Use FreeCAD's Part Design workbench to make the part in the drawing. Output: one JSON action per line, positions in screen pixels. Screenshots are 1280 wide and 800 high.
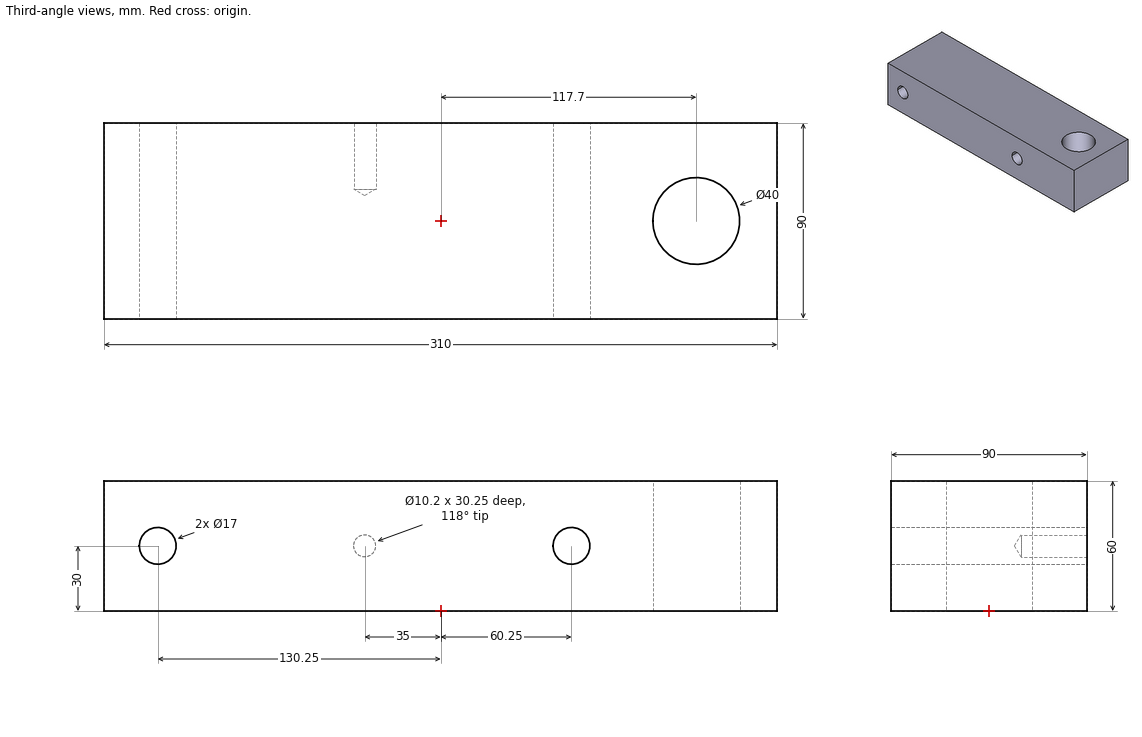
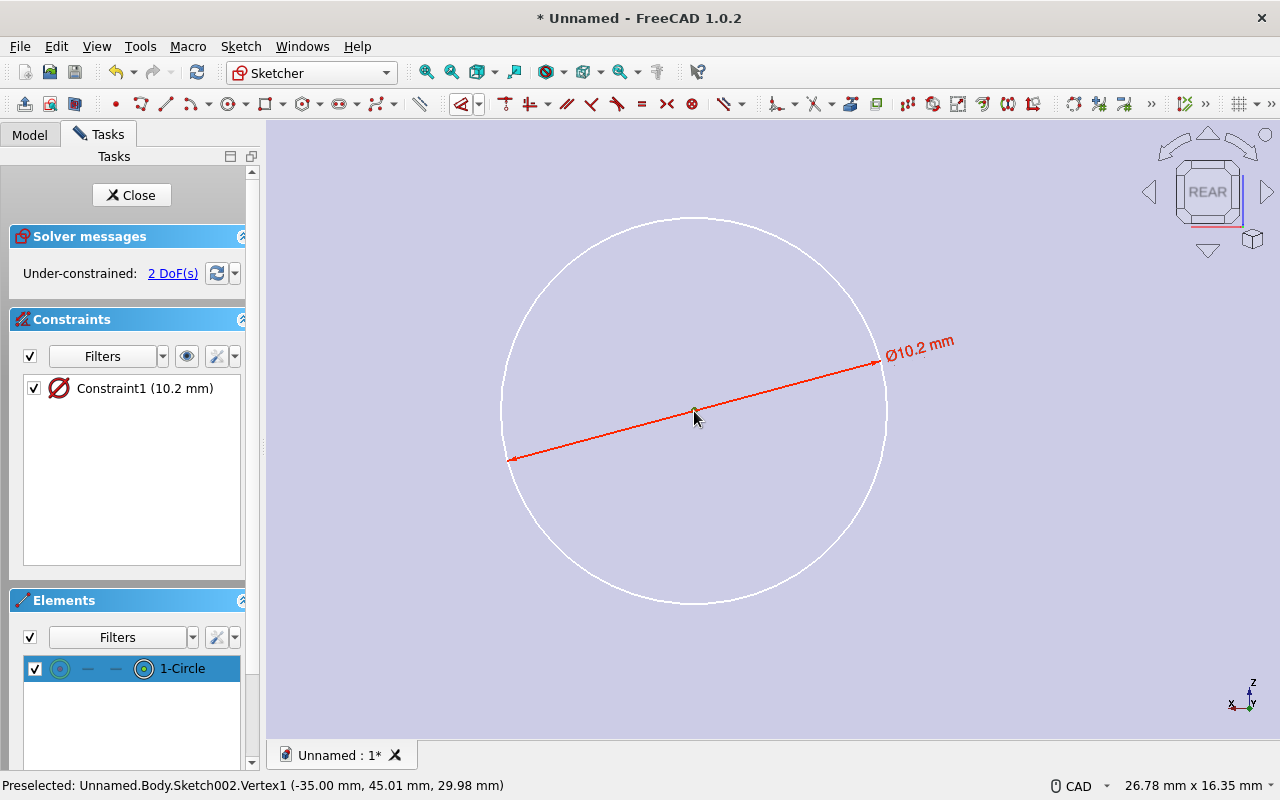
{"action": "key", "text": "l"}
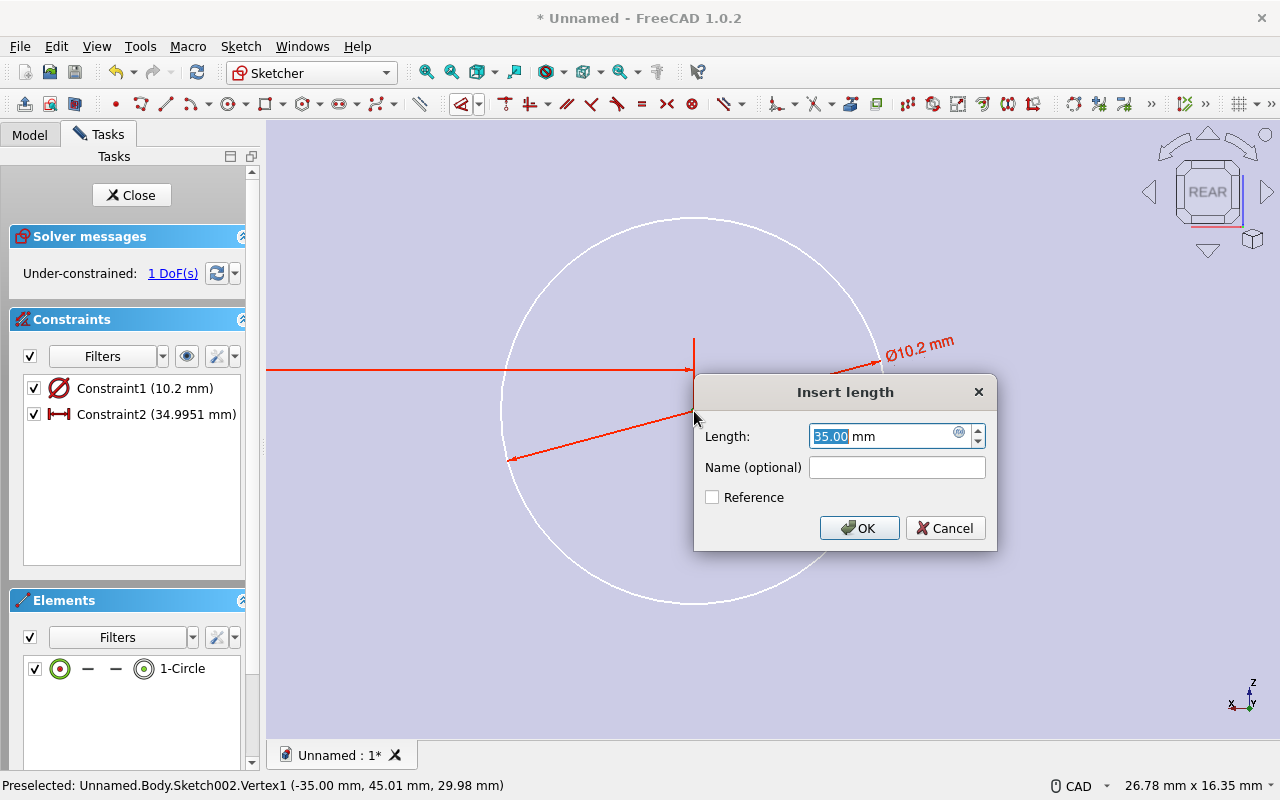
{"action": "type", "text": "35"}
{"action": "key", "text": "Return"}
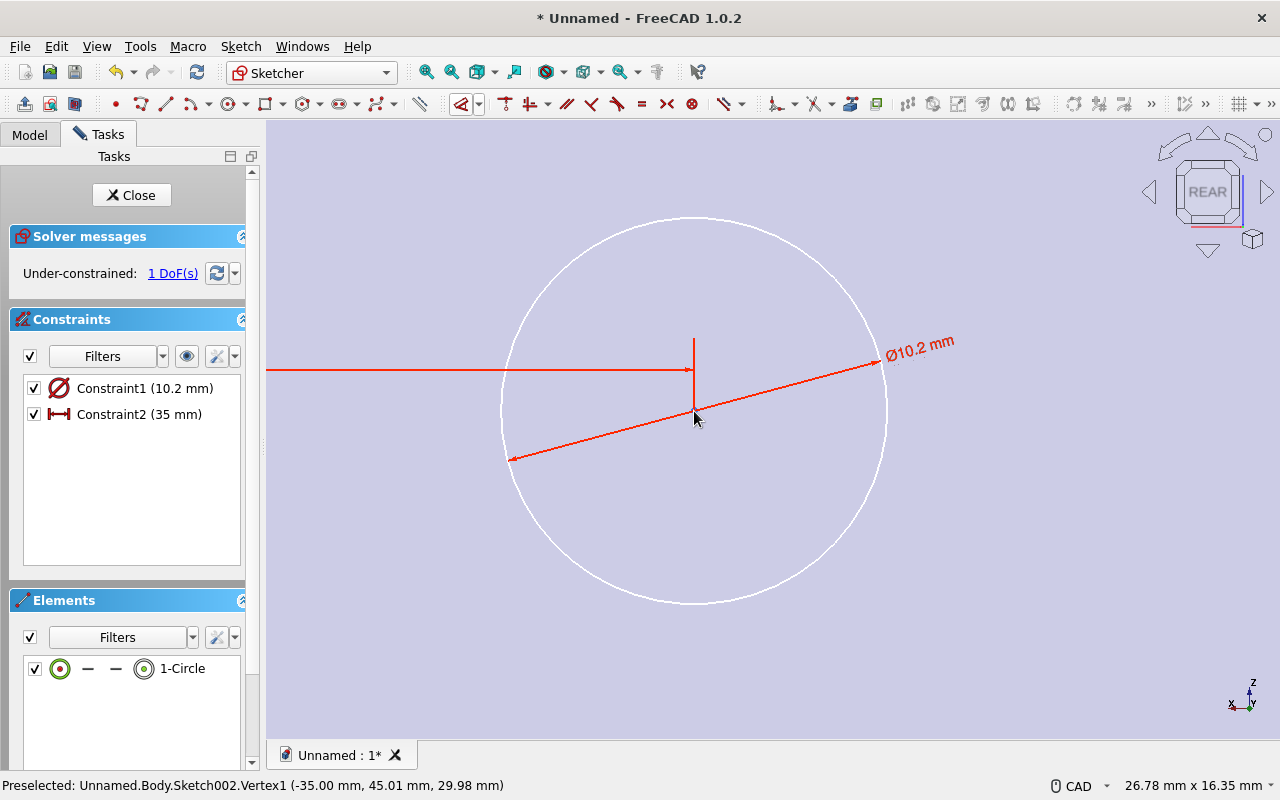
{"action": "left_click", "coordinate": [694, 411]}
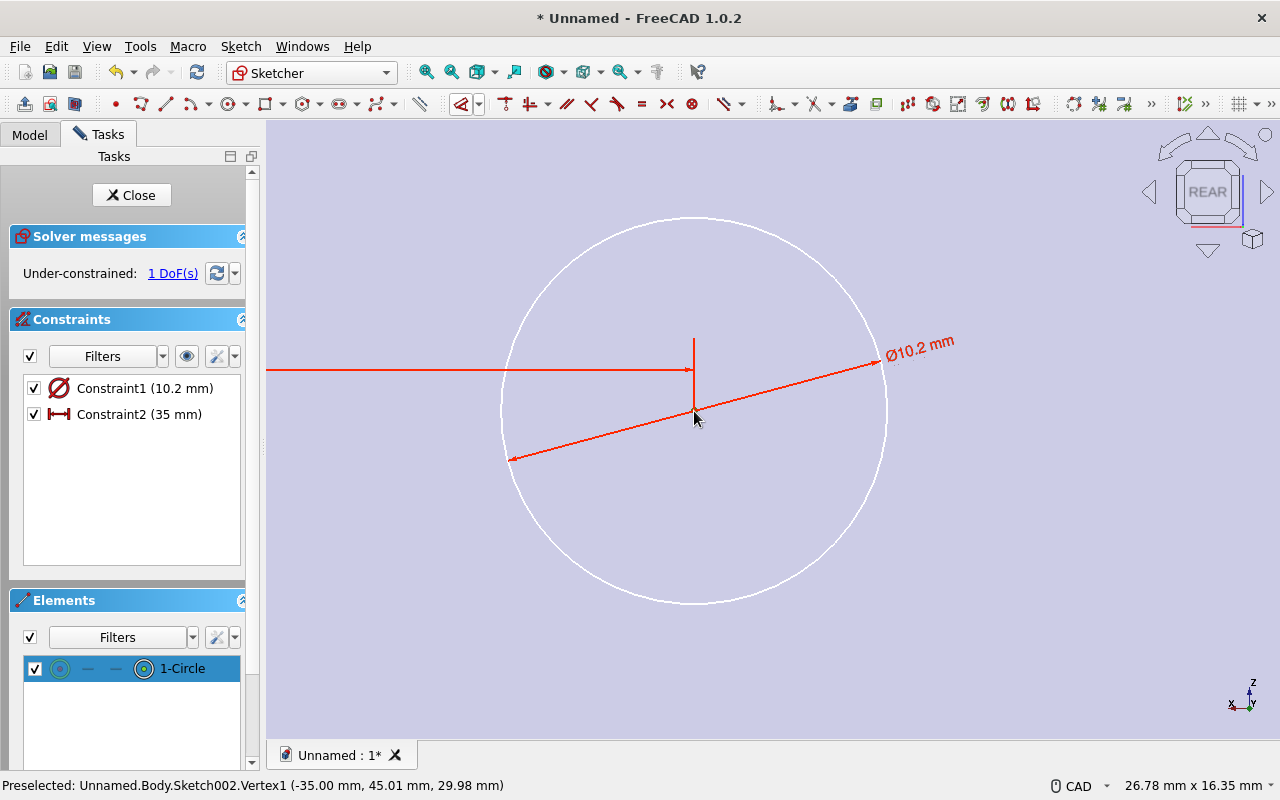
{"action": "left_click", "coordinate": [478, 104]}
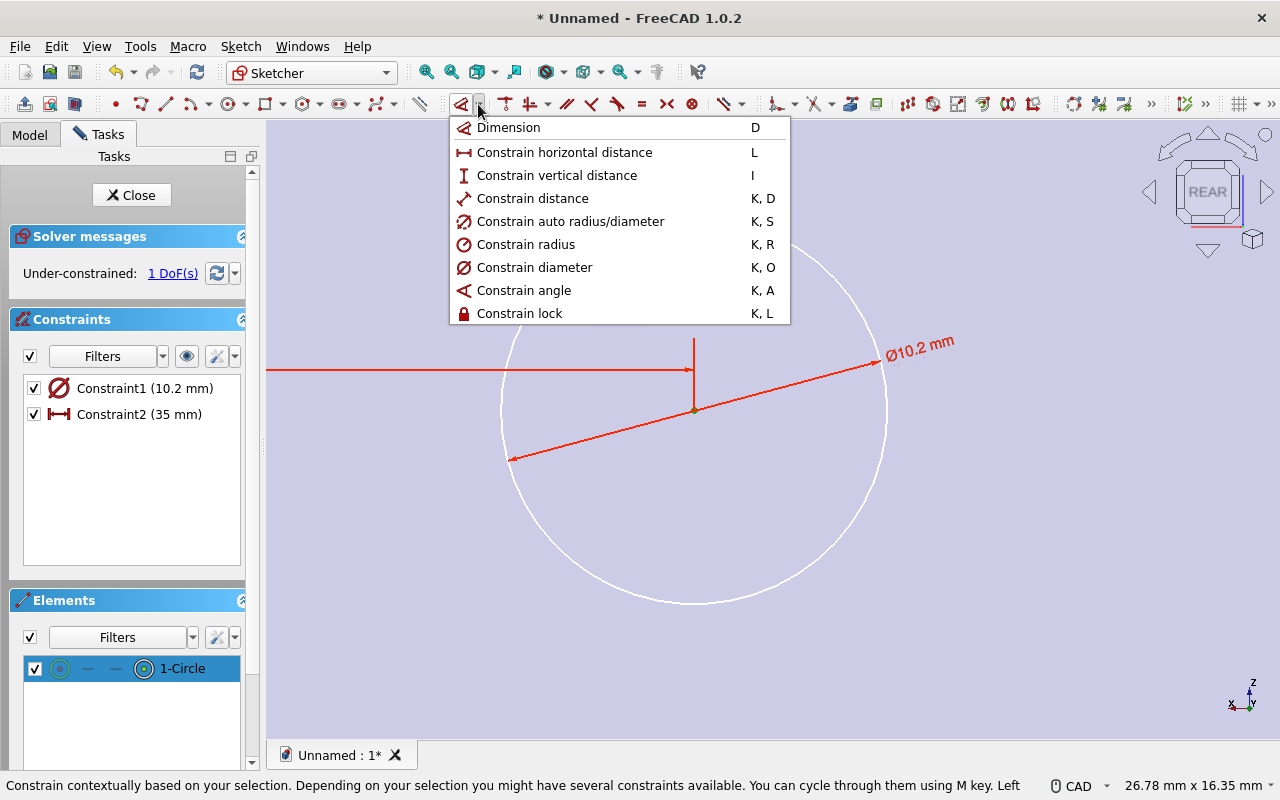
{"action": "left_click", "coordinate": [620, 176]}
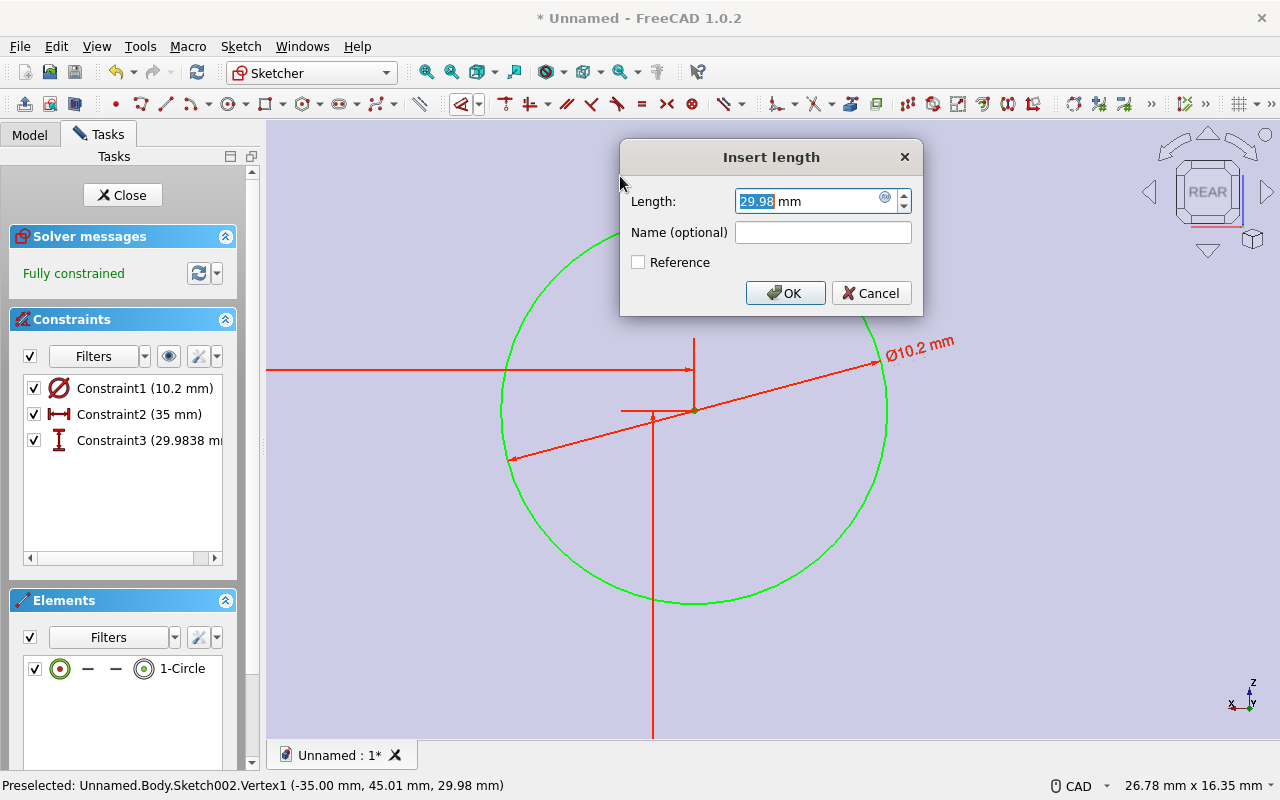
{"action": "type", "text": "30"}
{"action": "key", "text": "Return"}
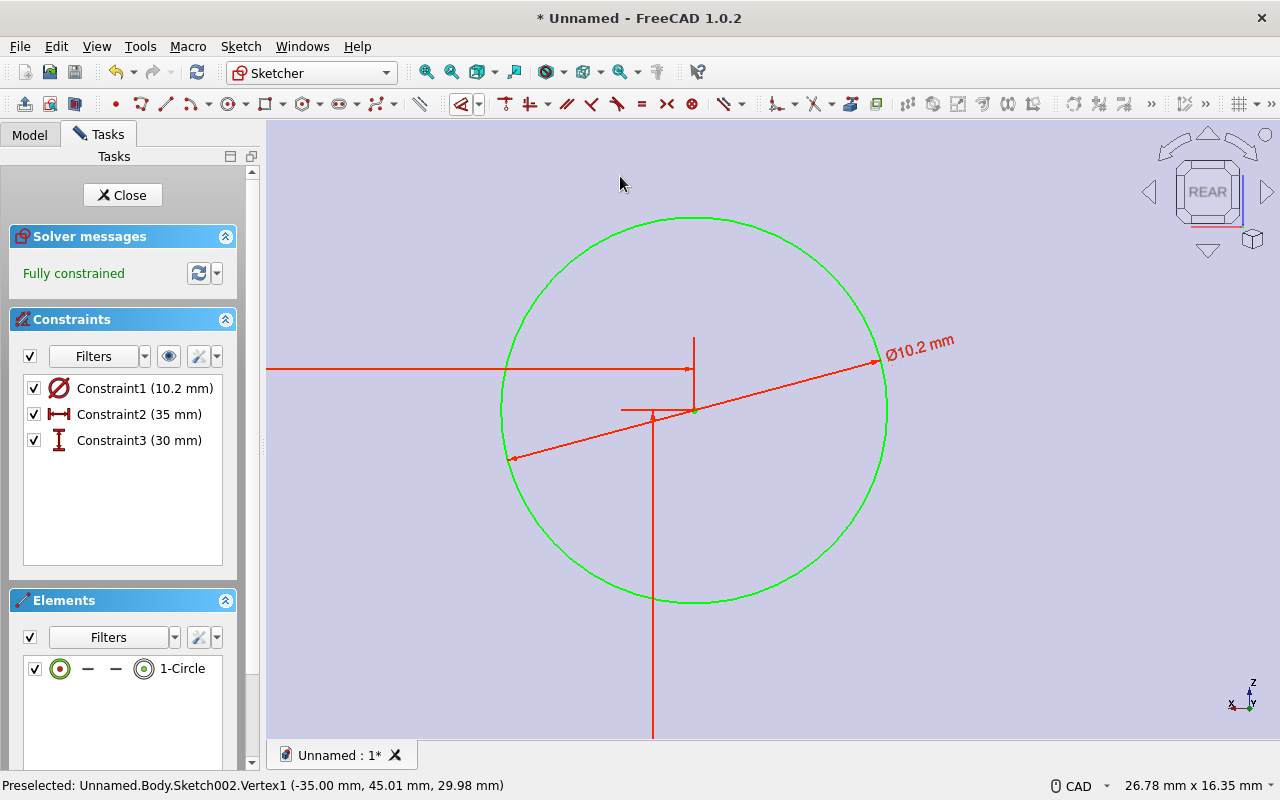
{"action": "left_click", "coordinate": [123, 195]}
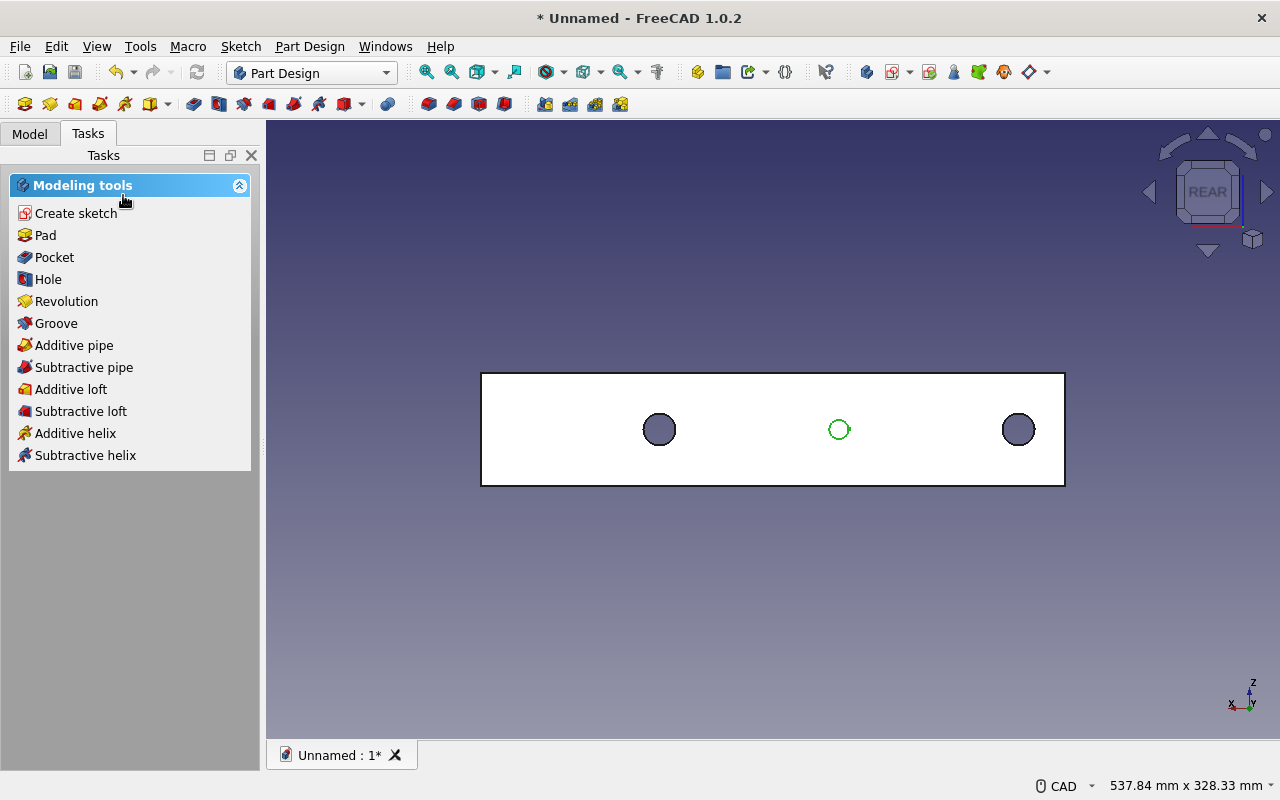
{"action": "left_click", "coordinate": [219, 104]}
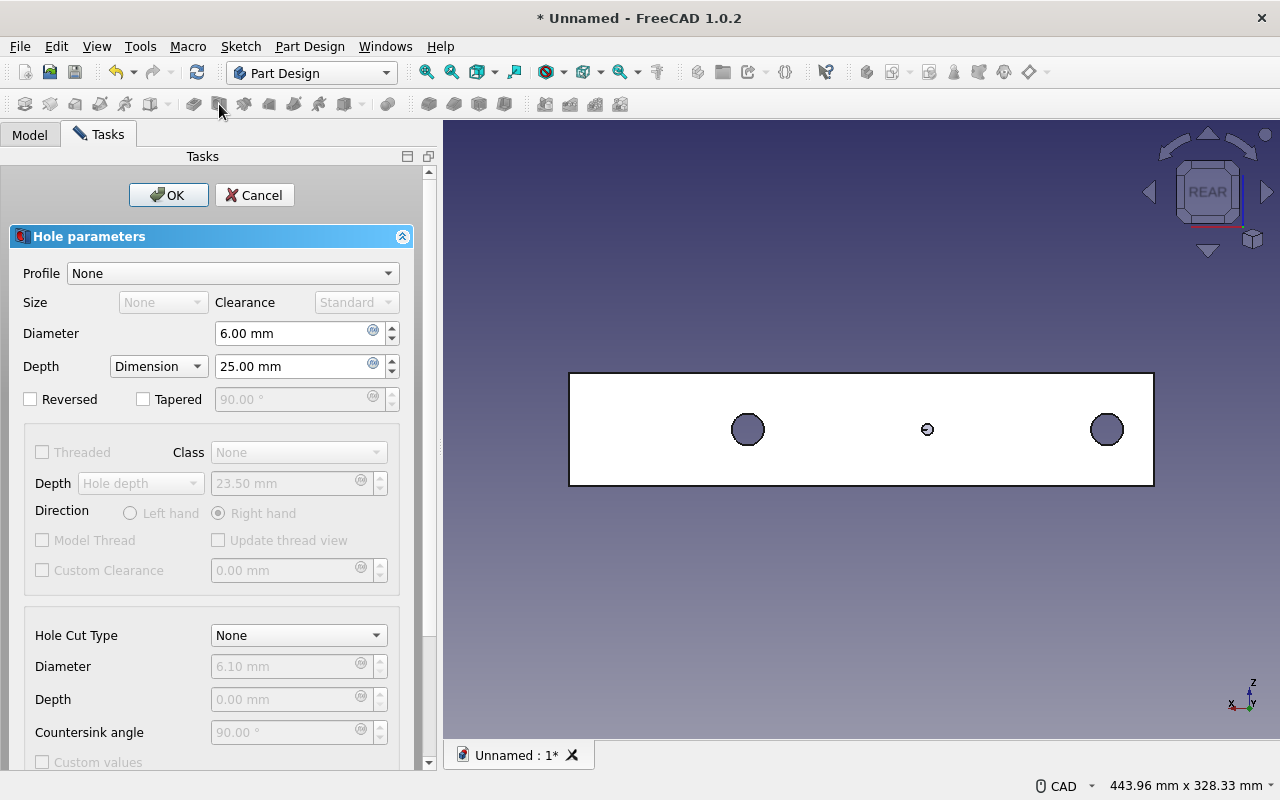
{"action": "triple_click", "coordinate": [300, 334]}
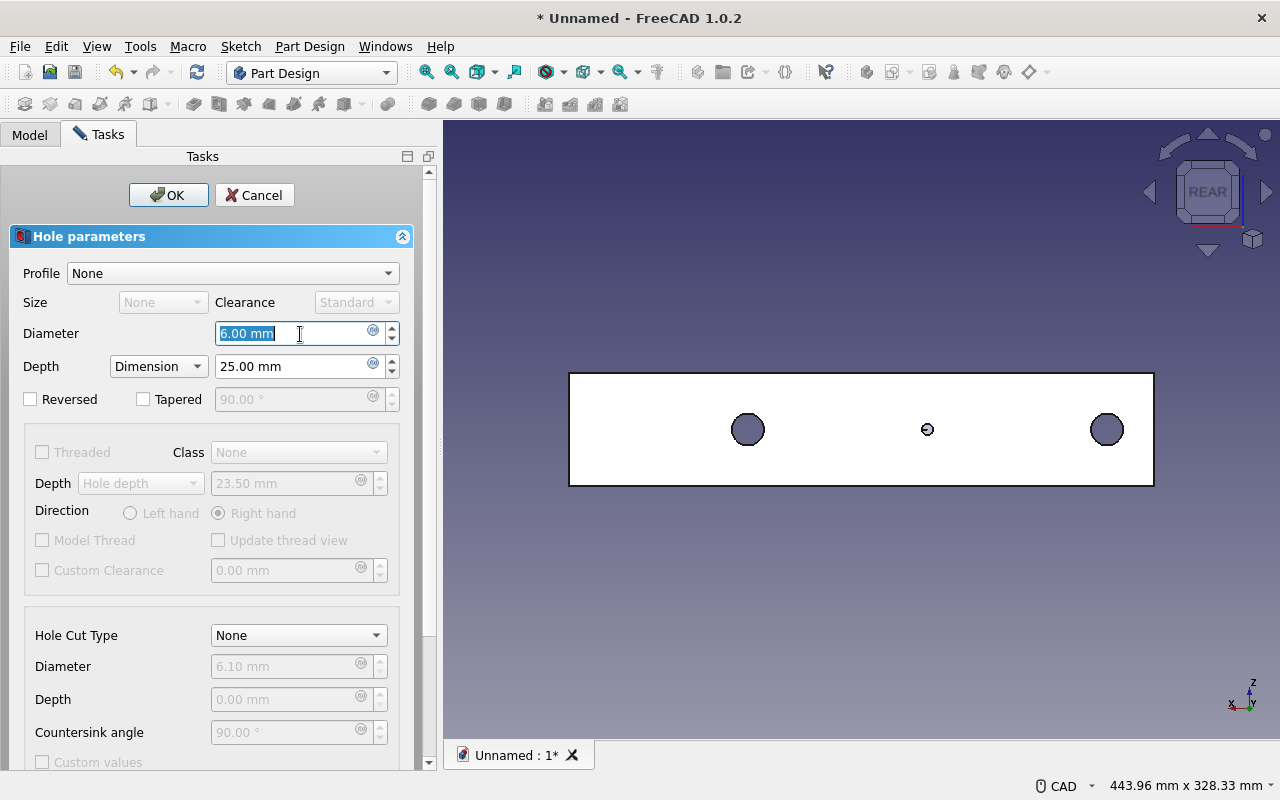
{"action": "type", "text": "10.2"}
{"action": "key", "text": "Tab"}